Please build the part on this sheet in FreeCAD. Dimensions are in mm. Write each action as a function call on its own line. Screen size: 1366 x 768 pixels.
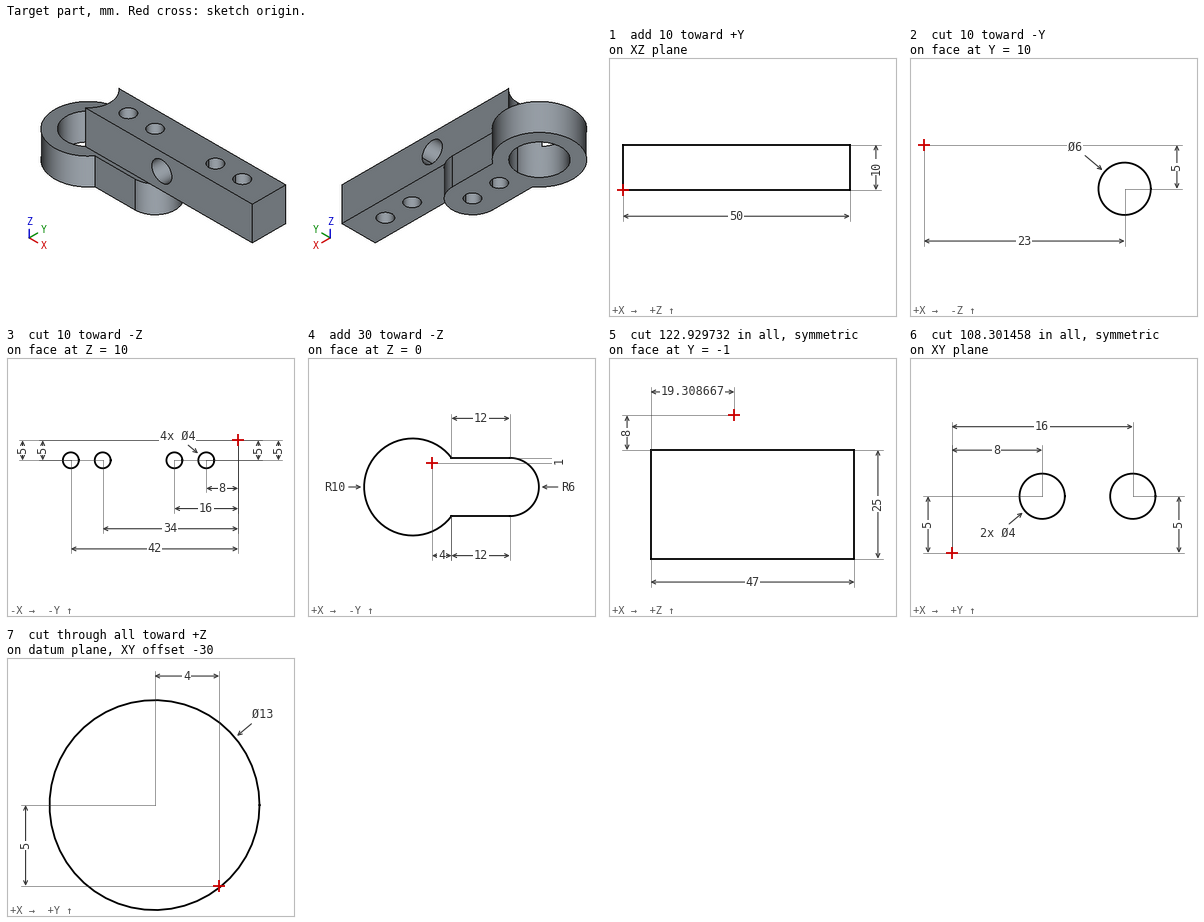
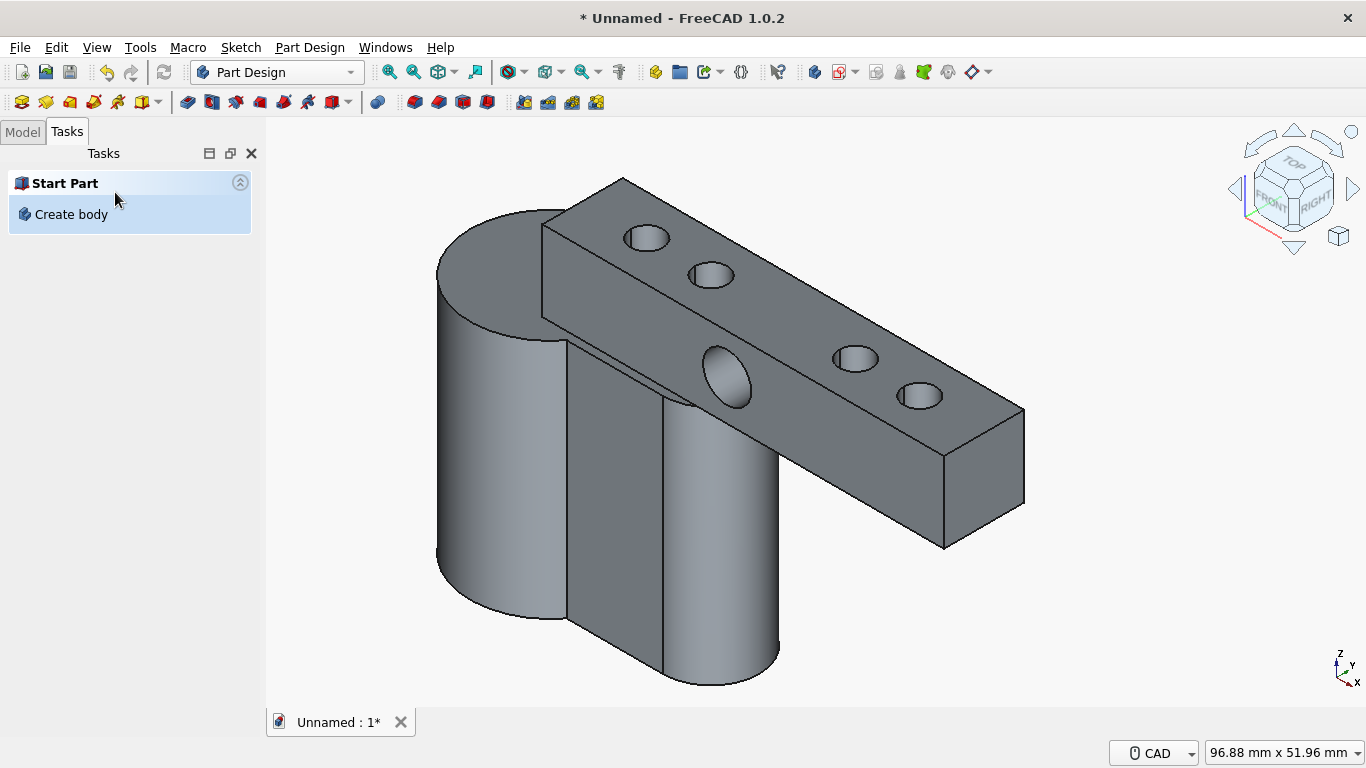
click(390, 72)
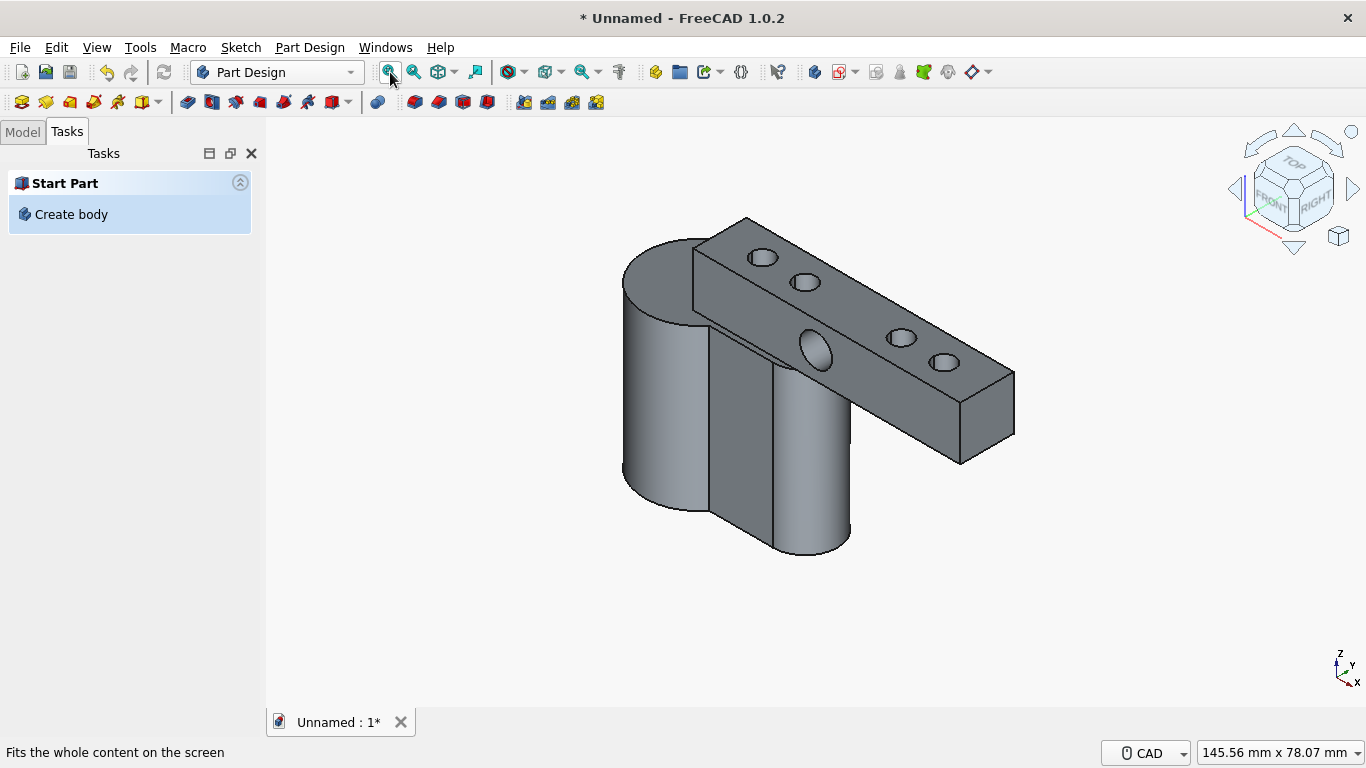
click(741, 383)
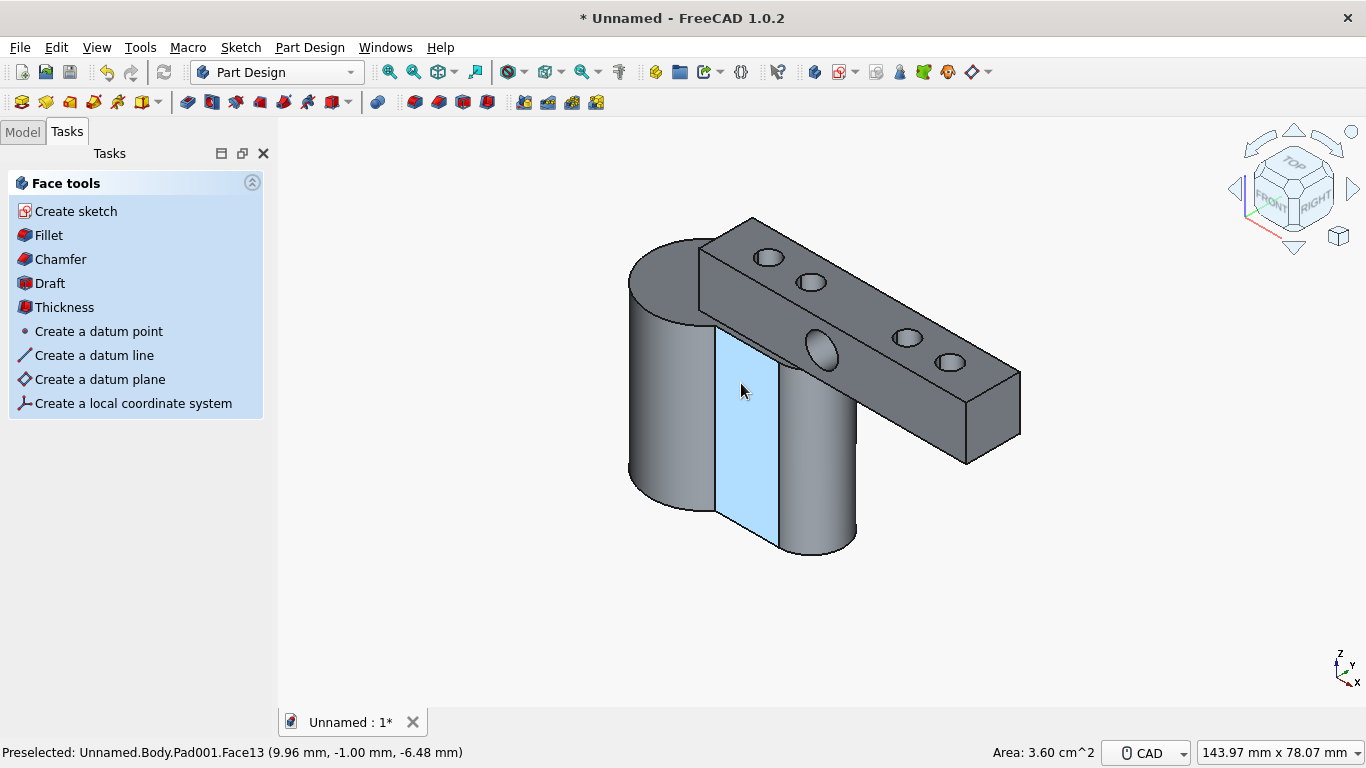
click(840, 72)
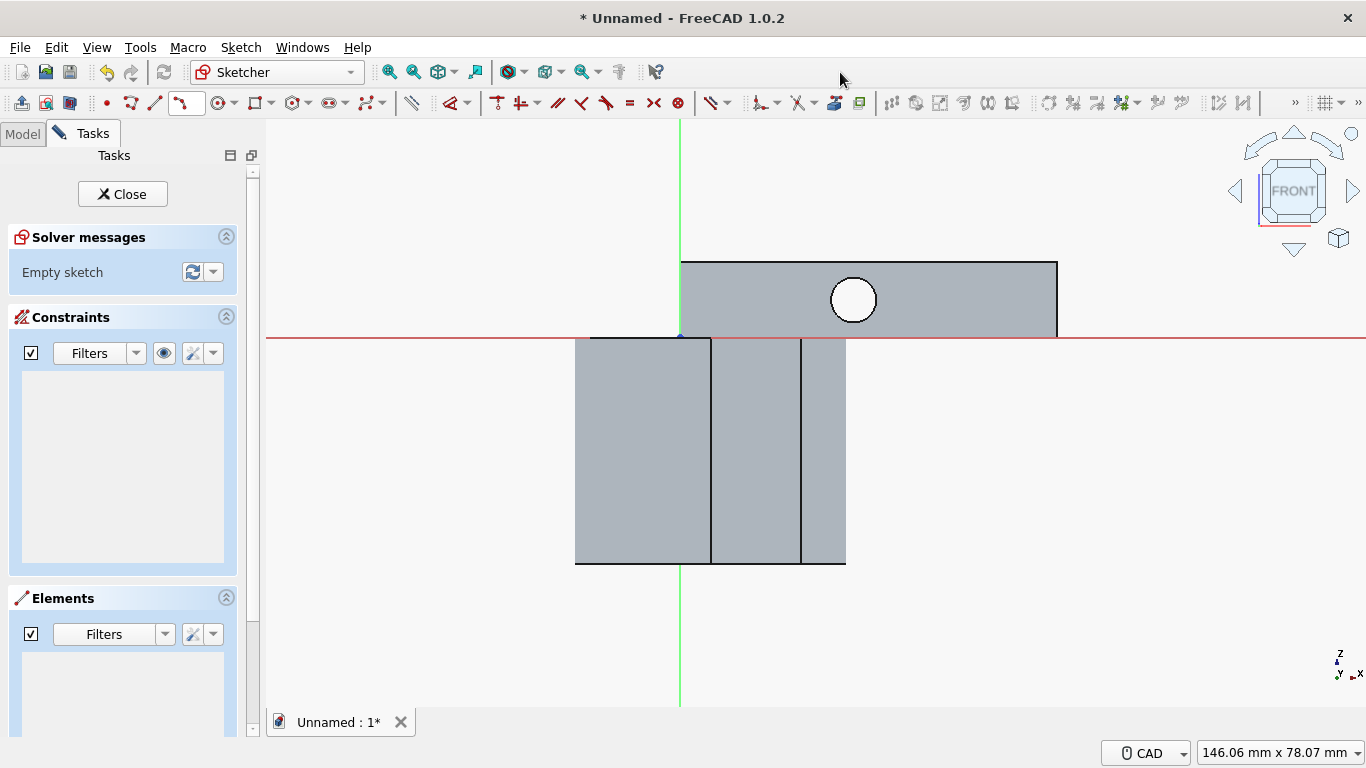
click(70, 104)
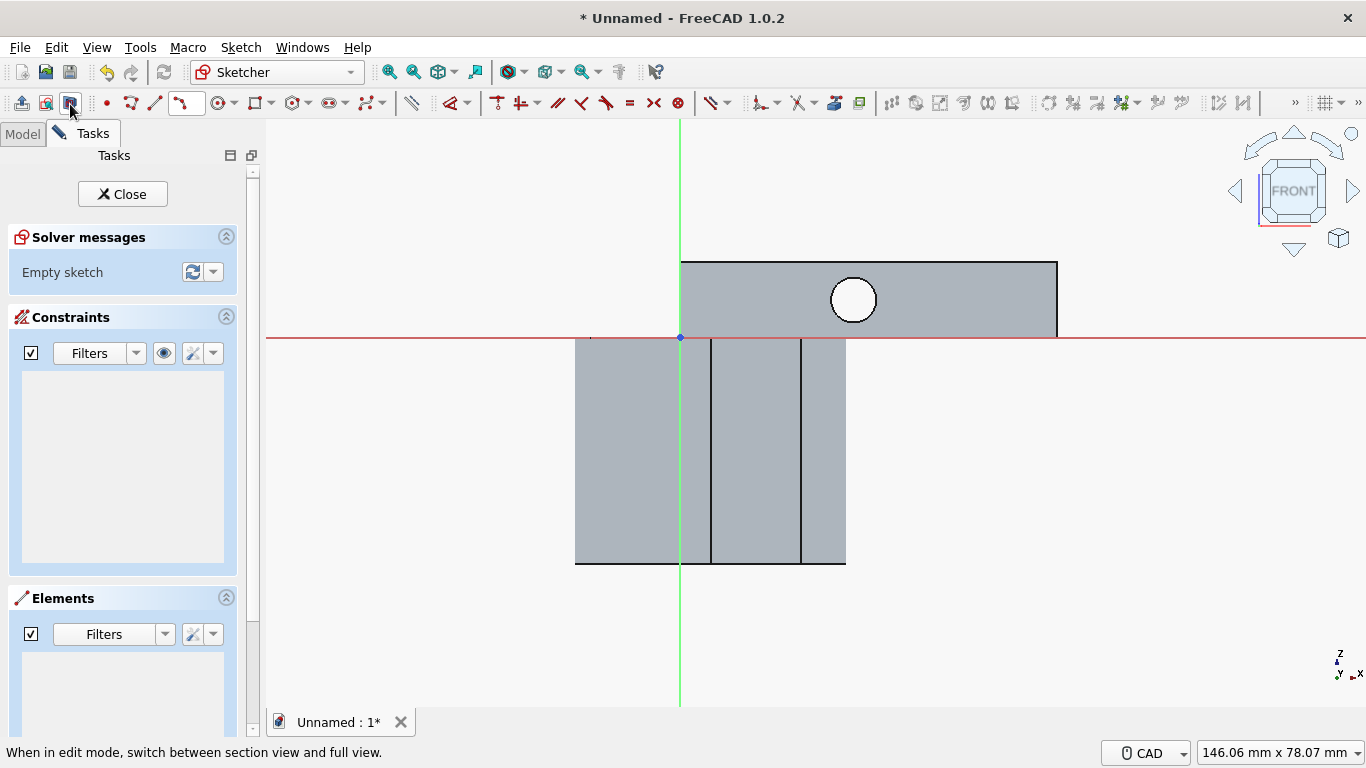
scroll(640, 561, up, 2)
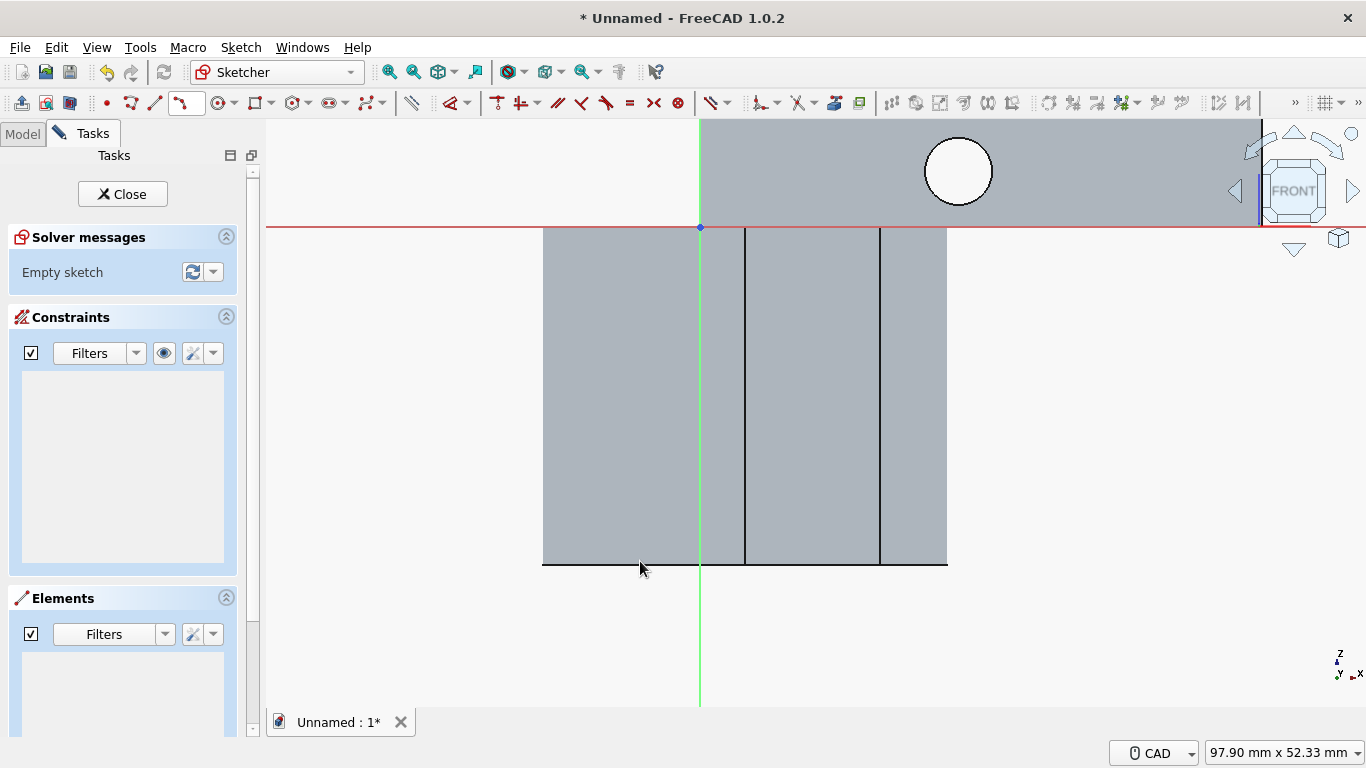
click(256, 104)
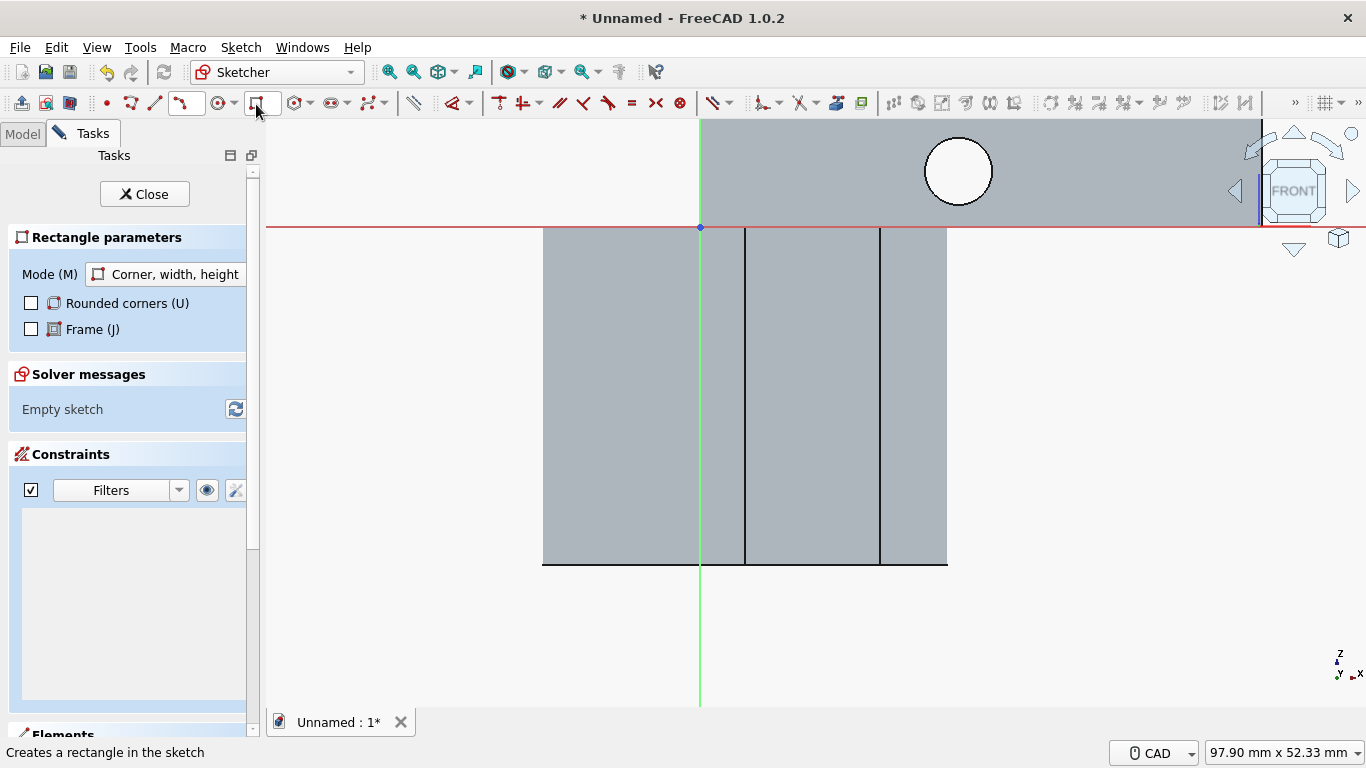
click(483, 317)
move(1011, 598)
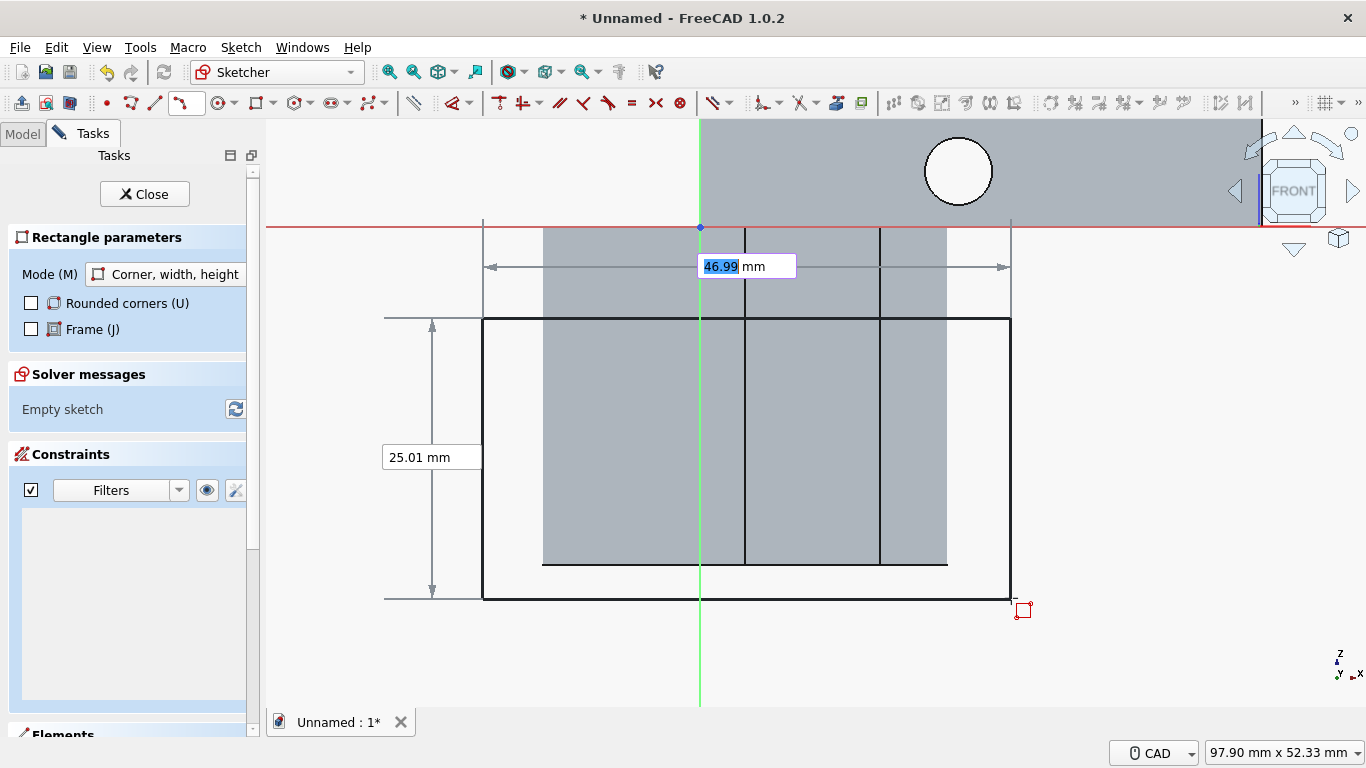
text(47)
key(Tab)
text(25)
key(Return)
key(Escape)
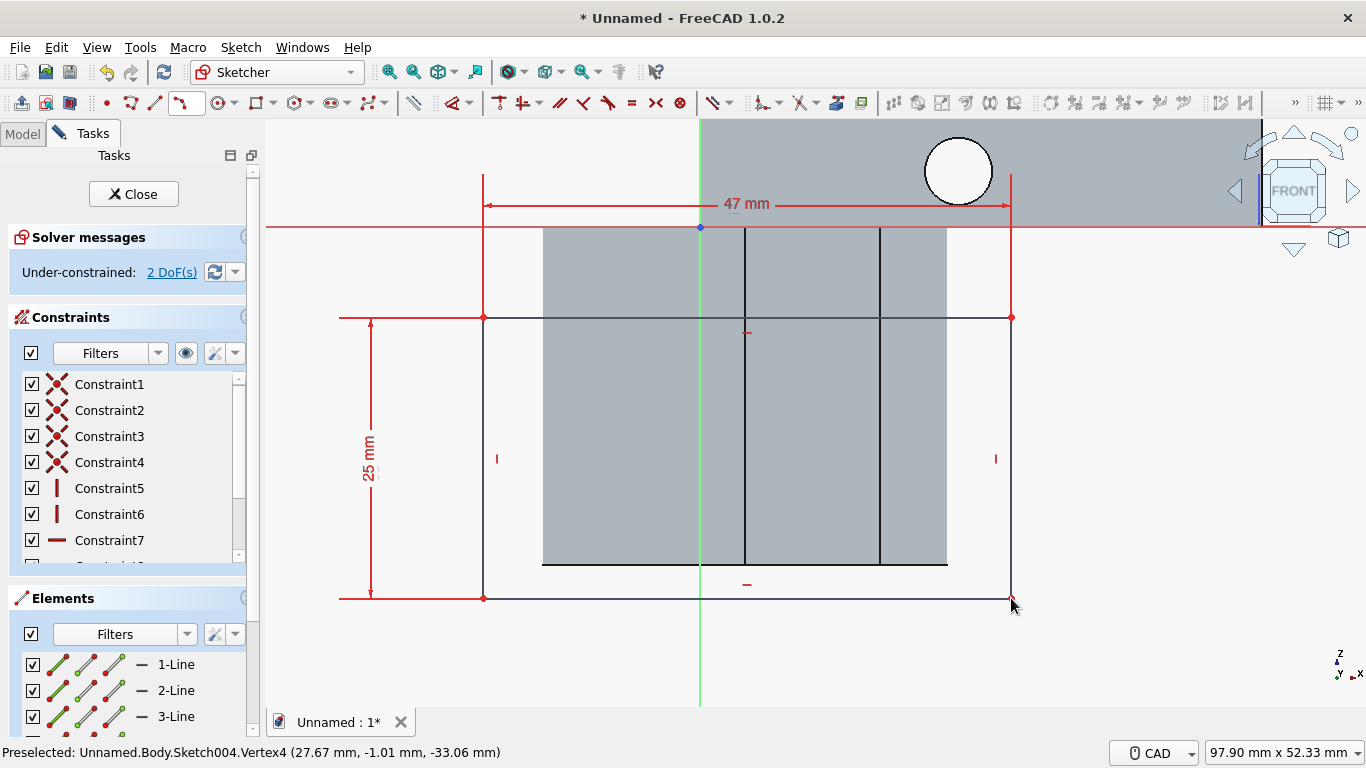
click(452, 104)